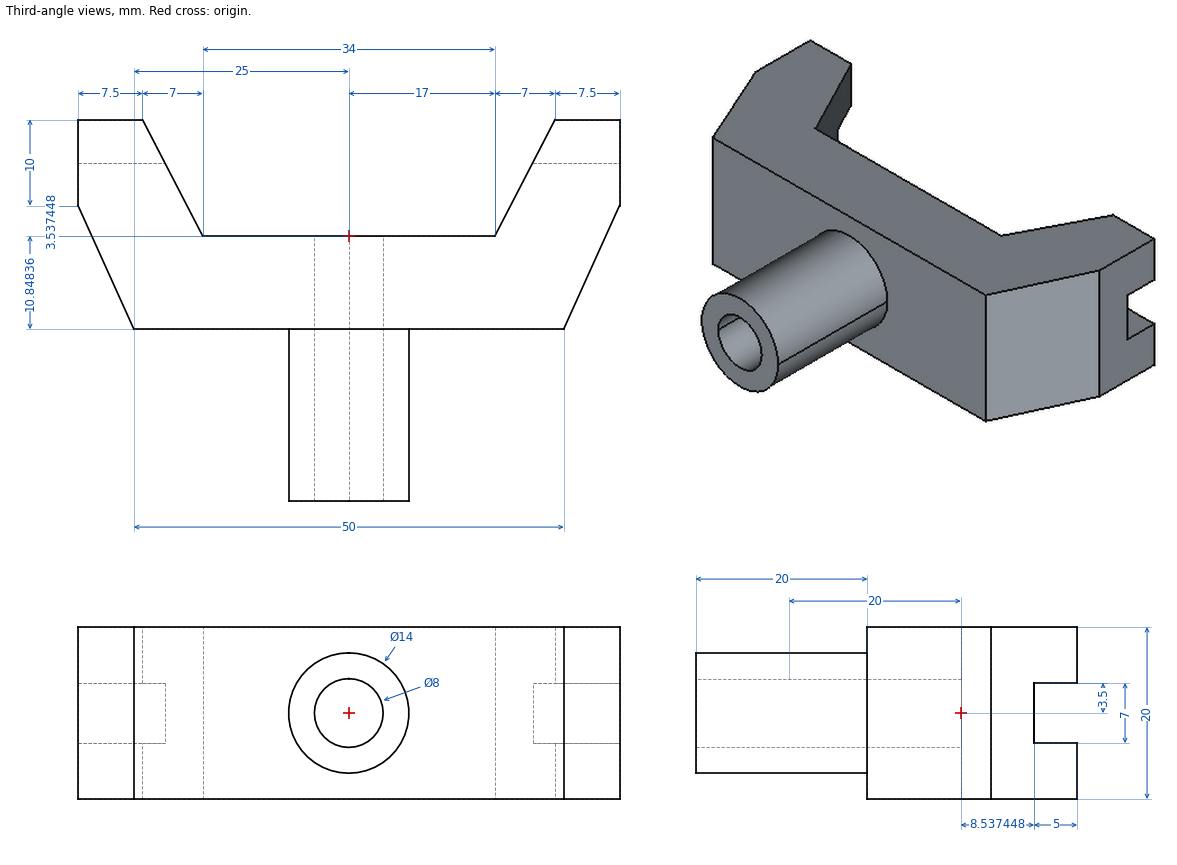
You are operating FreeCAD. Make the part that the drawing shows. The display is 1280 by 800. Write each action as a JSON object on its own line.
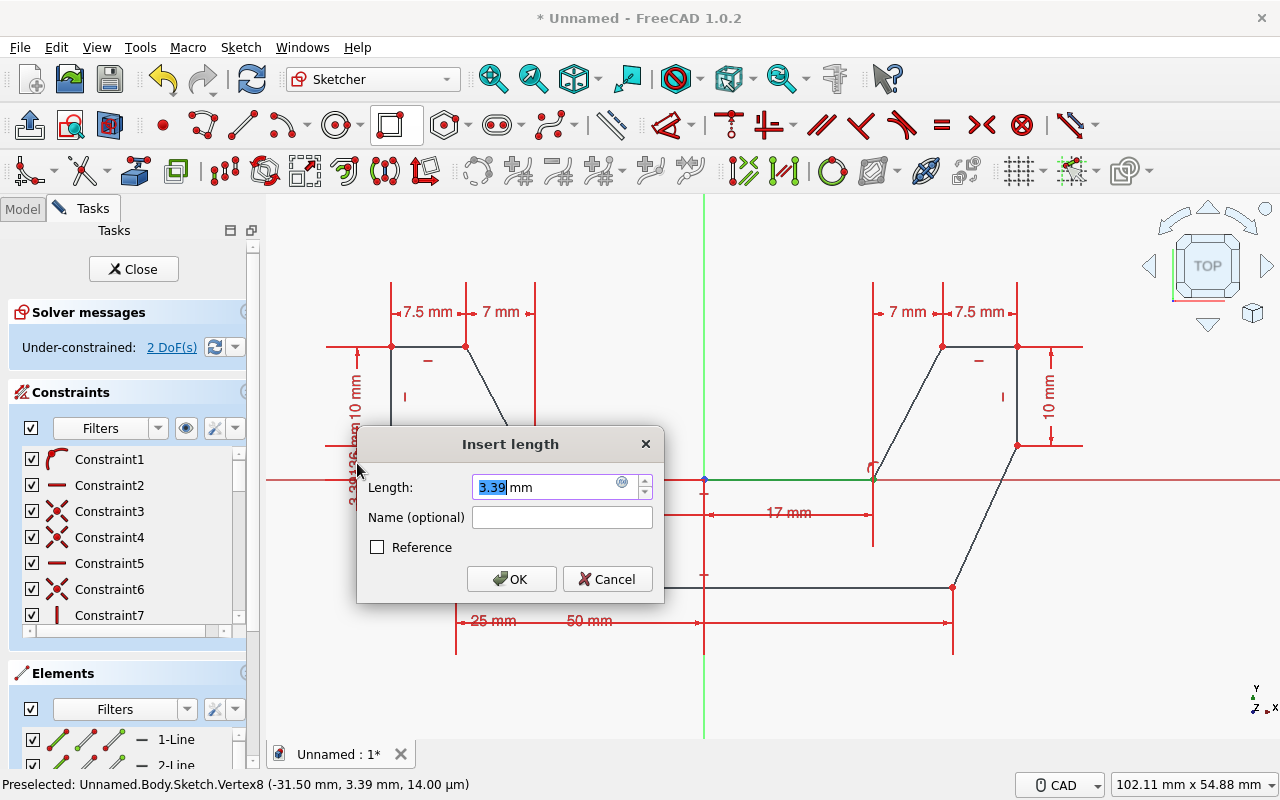
{"action": "type", "text": "3.537448"}
{"action": "key", "text": "Return"}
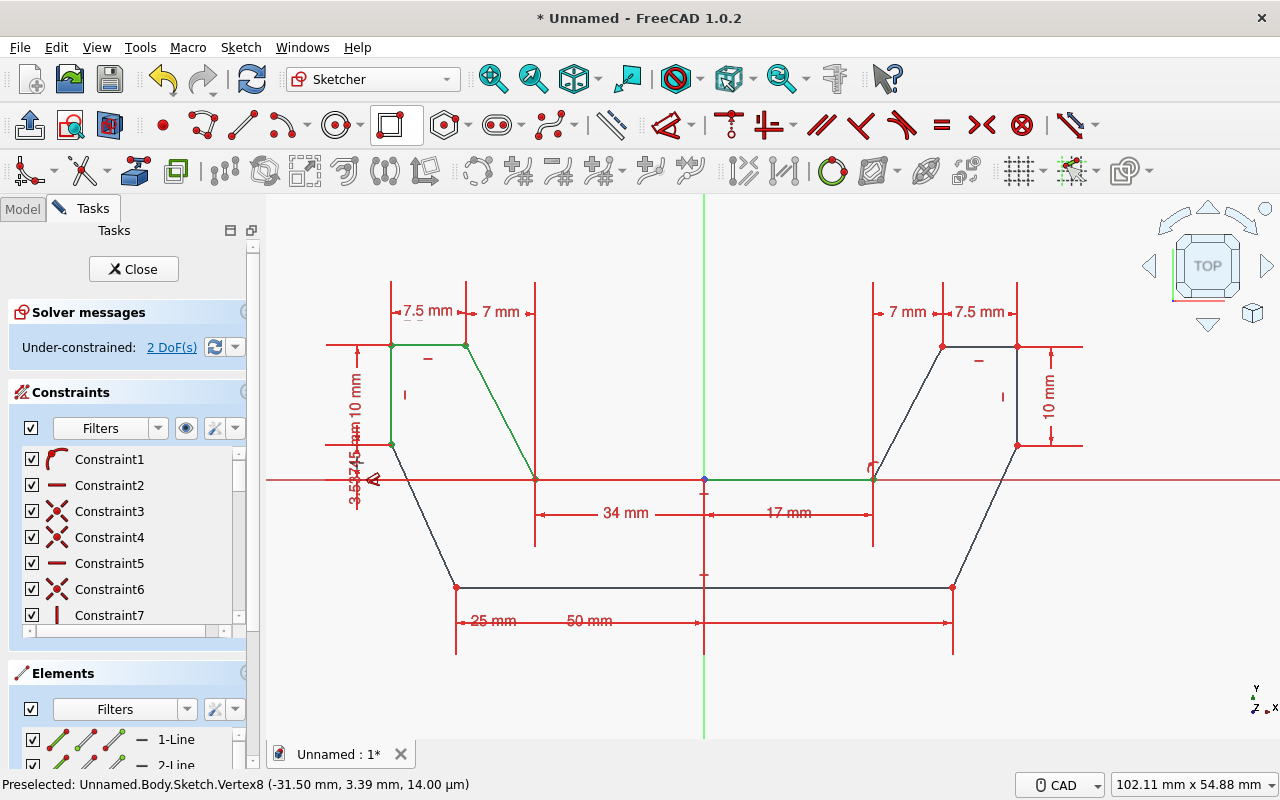
{"action": "left_click", "coordinate": [456, 588]}
{"action": "left_click", "coordinate": [422, 559]}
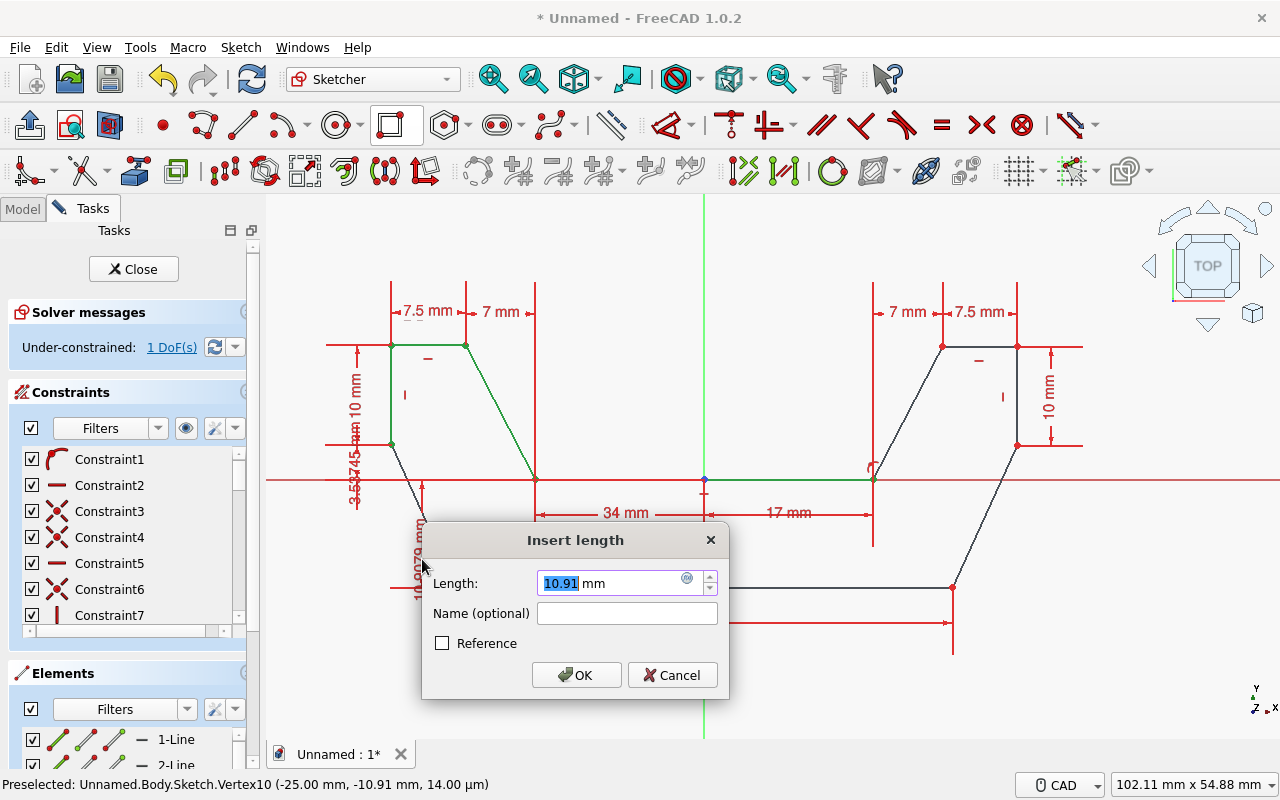
{"action": "type", "text": "10.84836"}
{"action": "key", "text": "Return"}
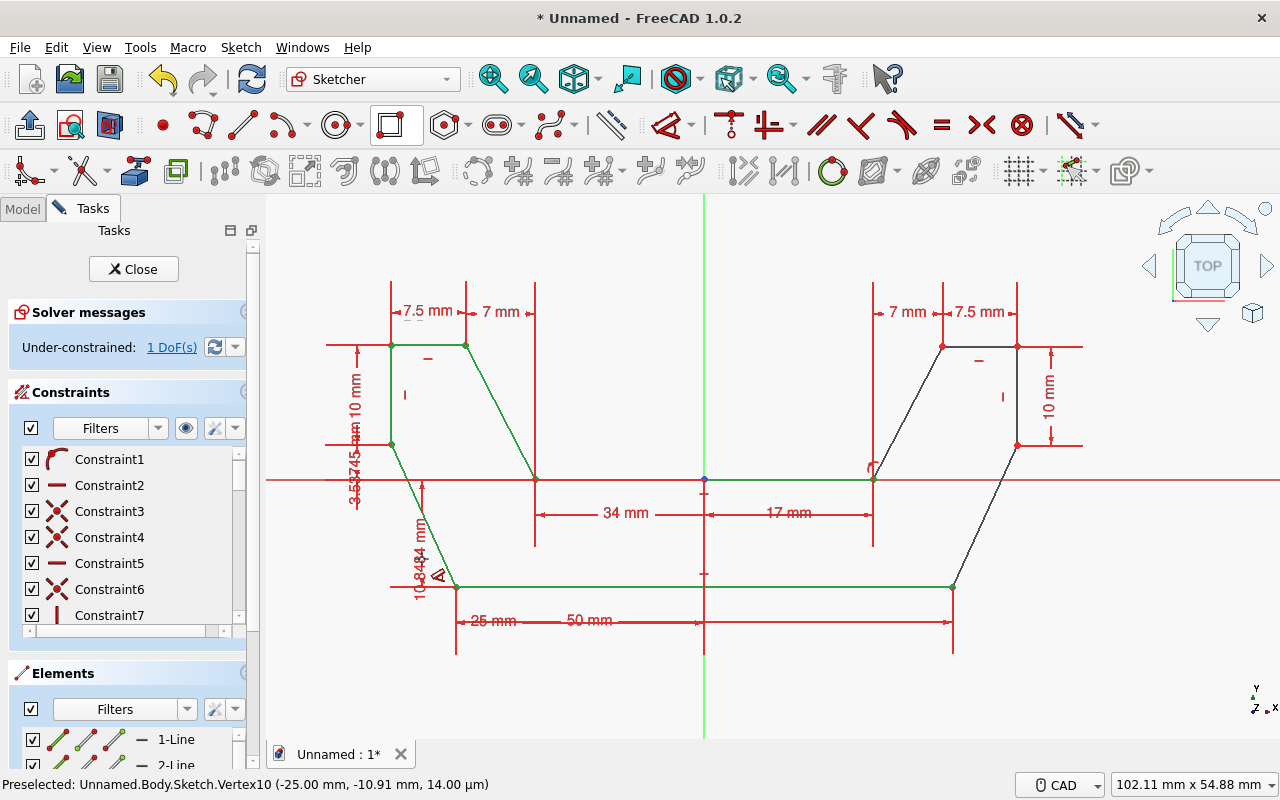
{"action": "left_click", "coordinate": [1017, 446]}
{"action": "left_click", "coordinate": [1051, 463]}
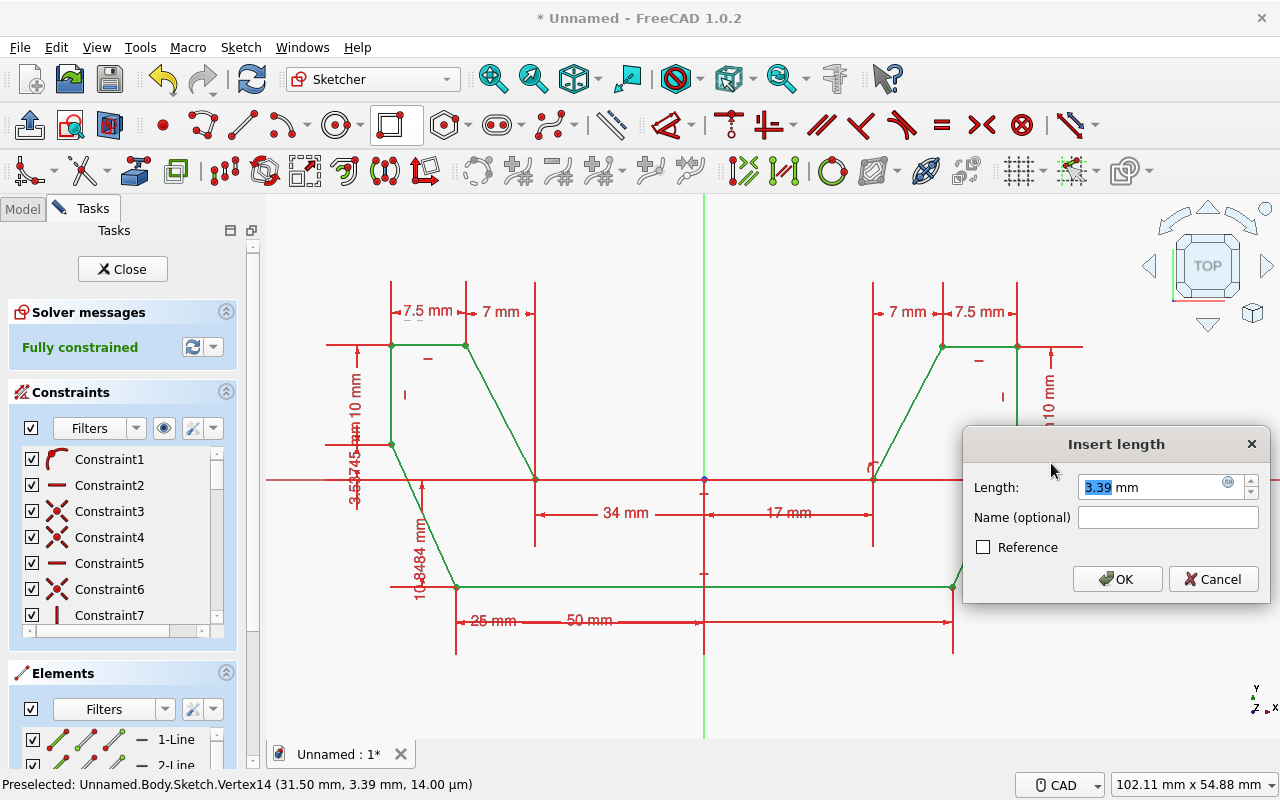
{"action": "type", "text": "3.537448"}
{"action": "key", "text": "Return"}
{"action": "key", "text": "Escape"}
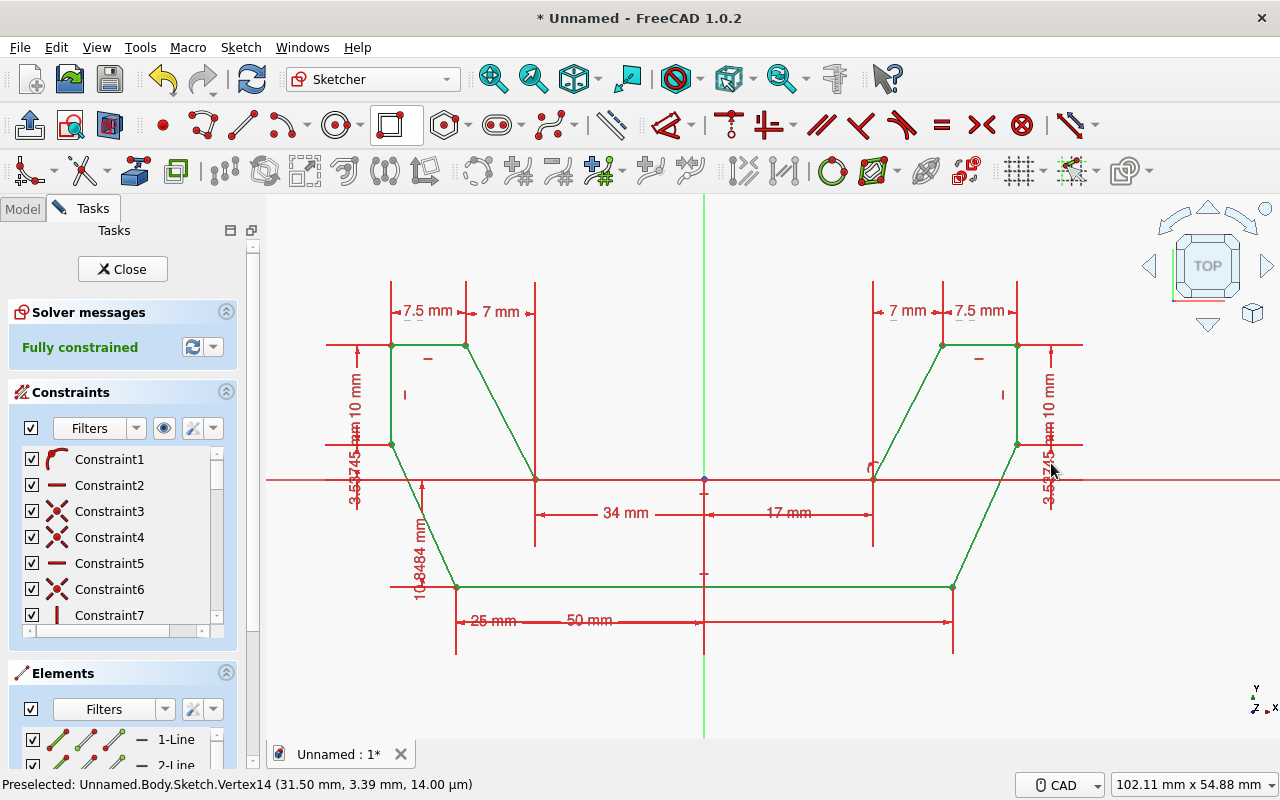
{"action": "left_click", "coordinate": [123, 269]}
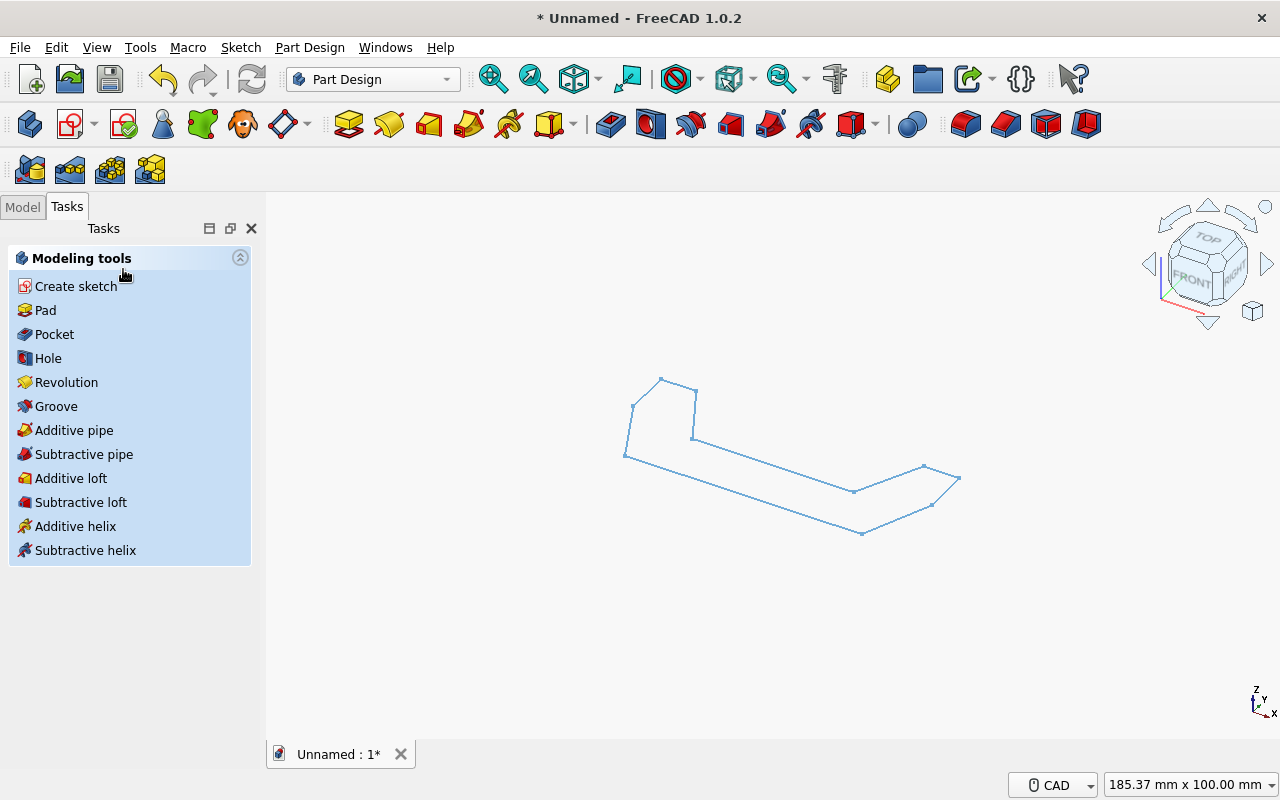
{"action": "left_click", "coordinate": [350, 124]}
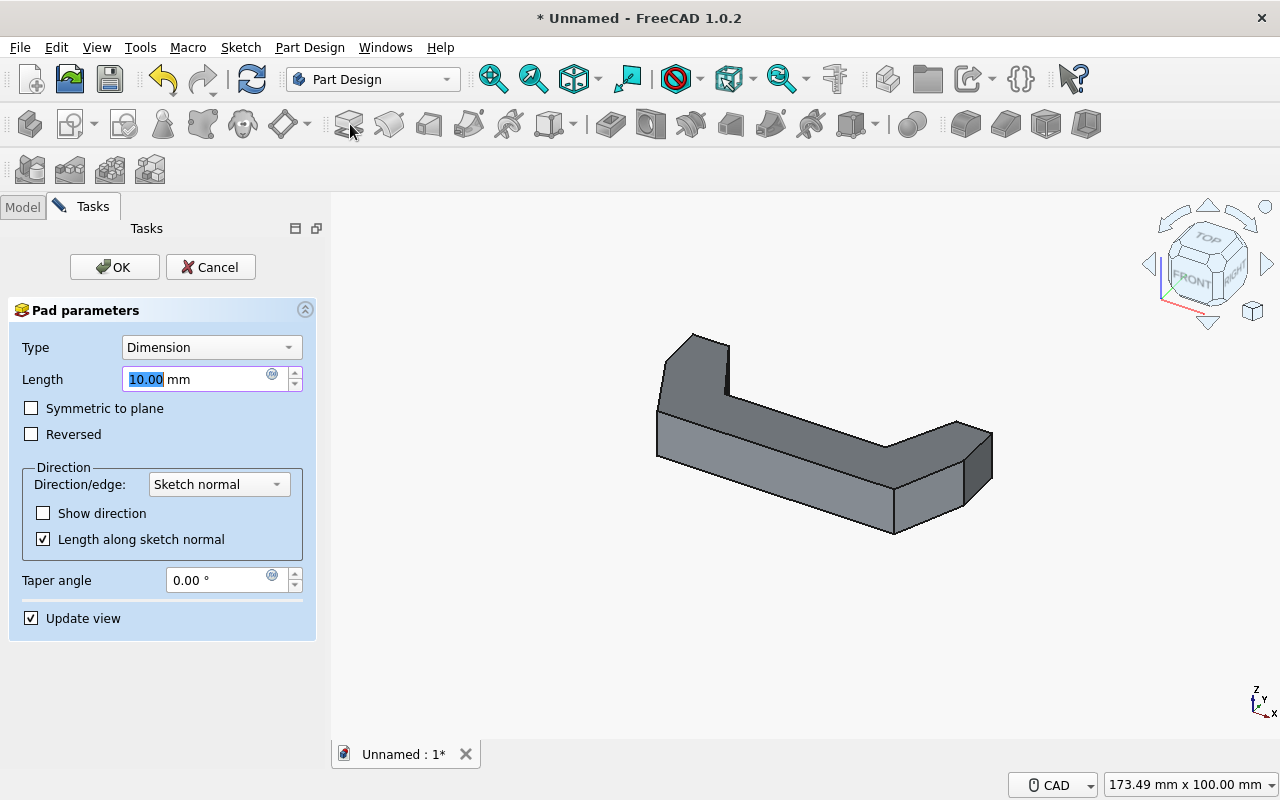
{"action": "type", "text": "20"}
{"action": "key", "text": "Tab"}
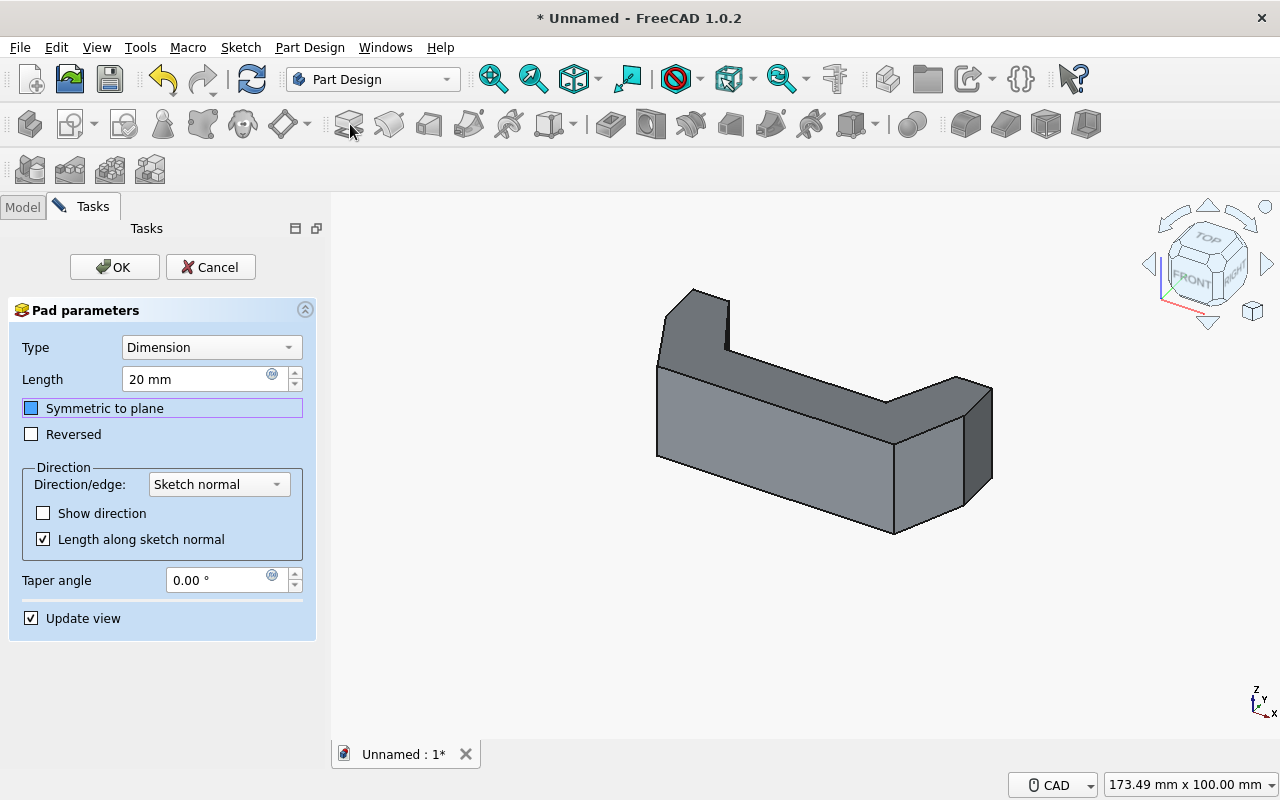
{"action": "left_click", "coordinate": [30, 408]}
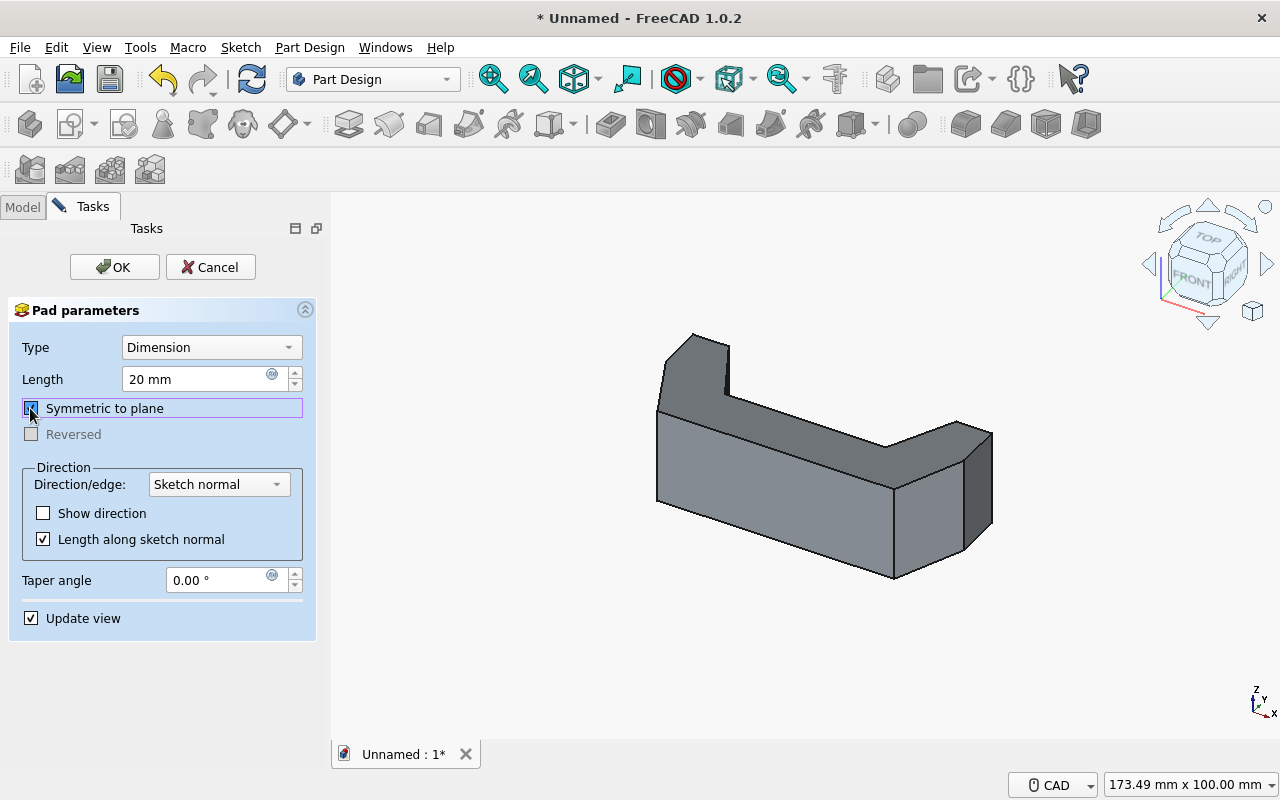
{"action": "left_click", "coordinate": [115, 267]}